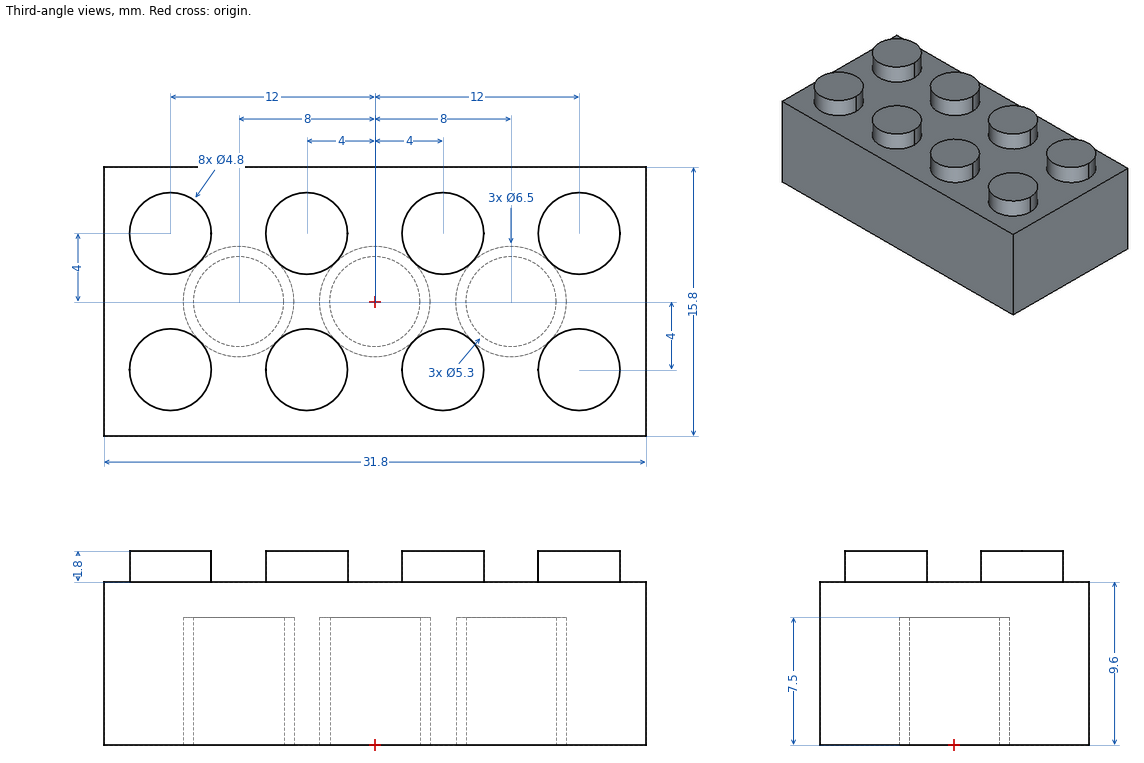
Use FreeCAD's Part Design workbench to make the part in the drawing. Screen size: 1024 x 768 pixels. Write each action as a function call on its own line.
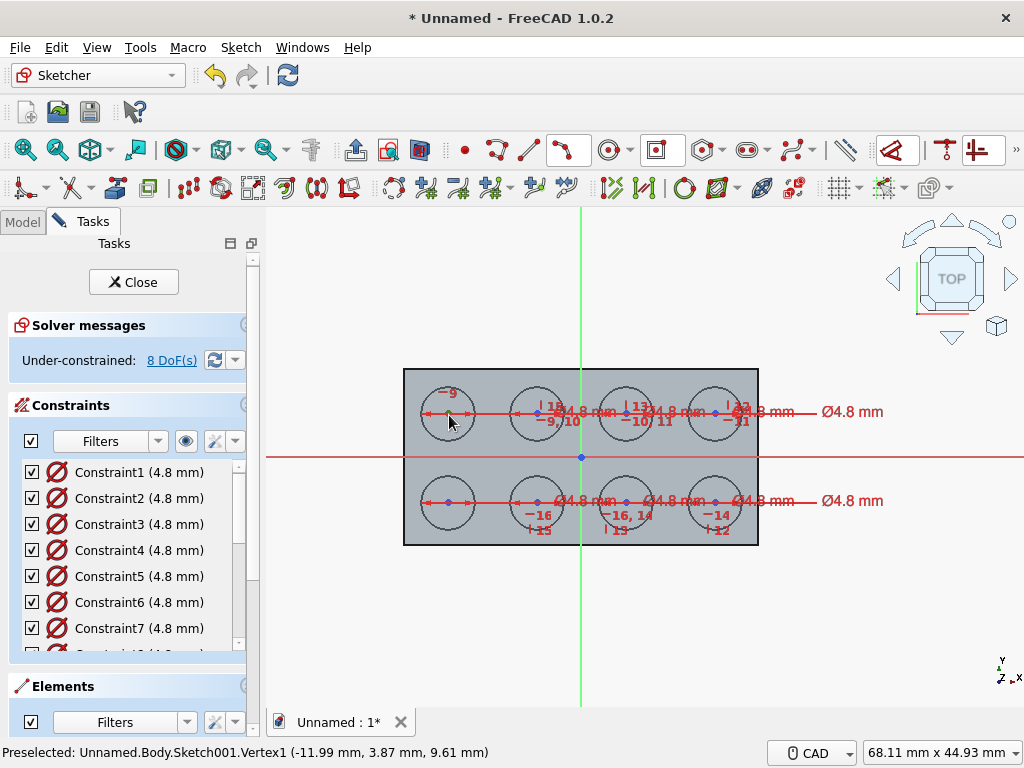
click(448, 503)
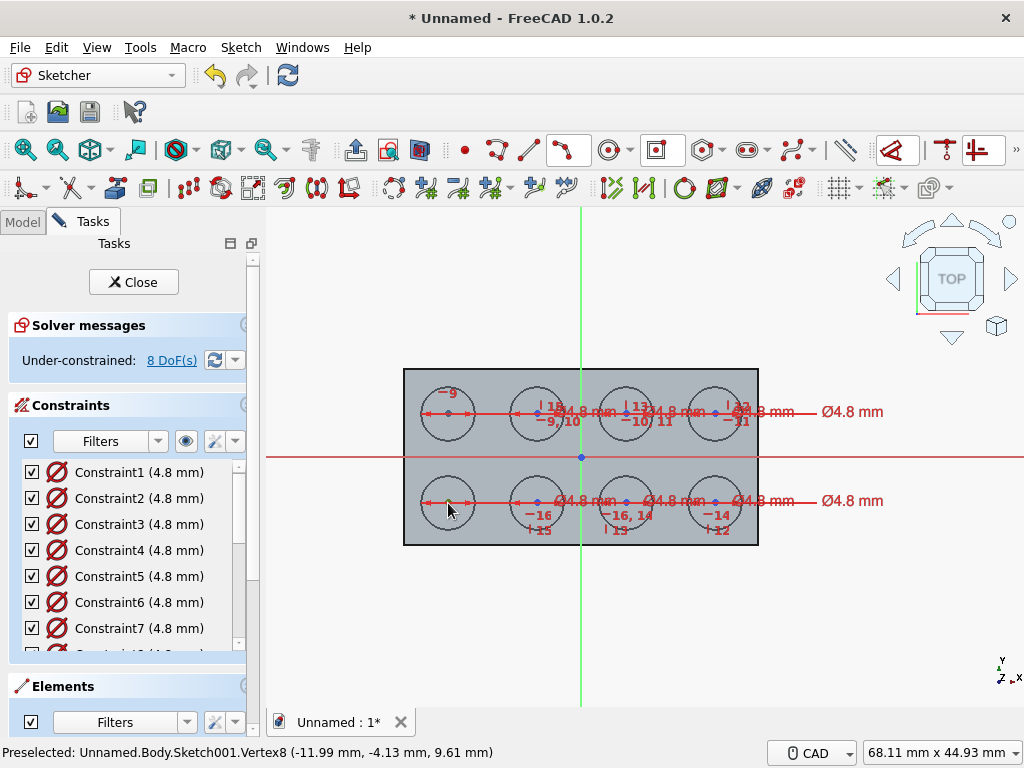
click(1000, 150)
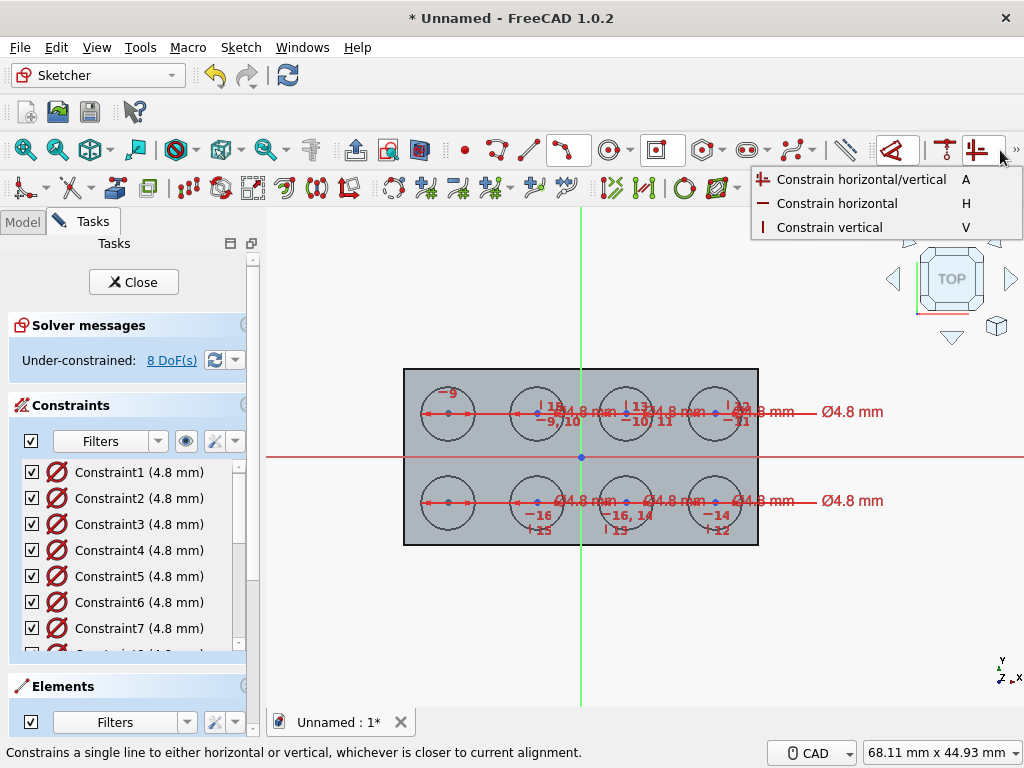
click(887, 227)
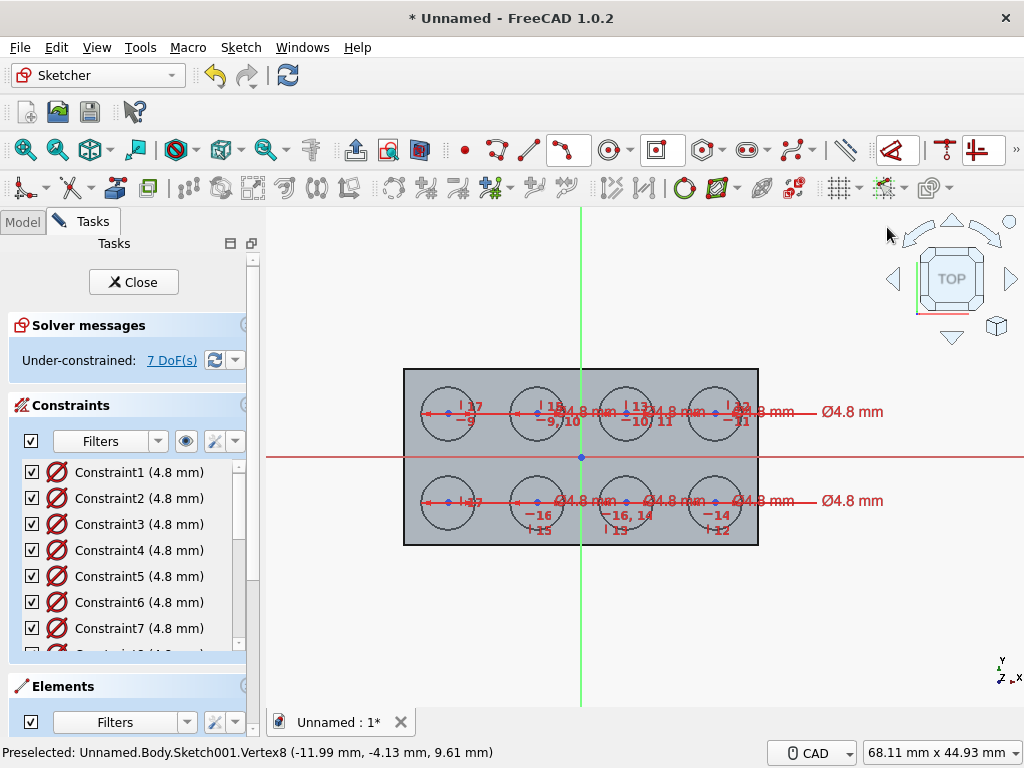
click(537, 503)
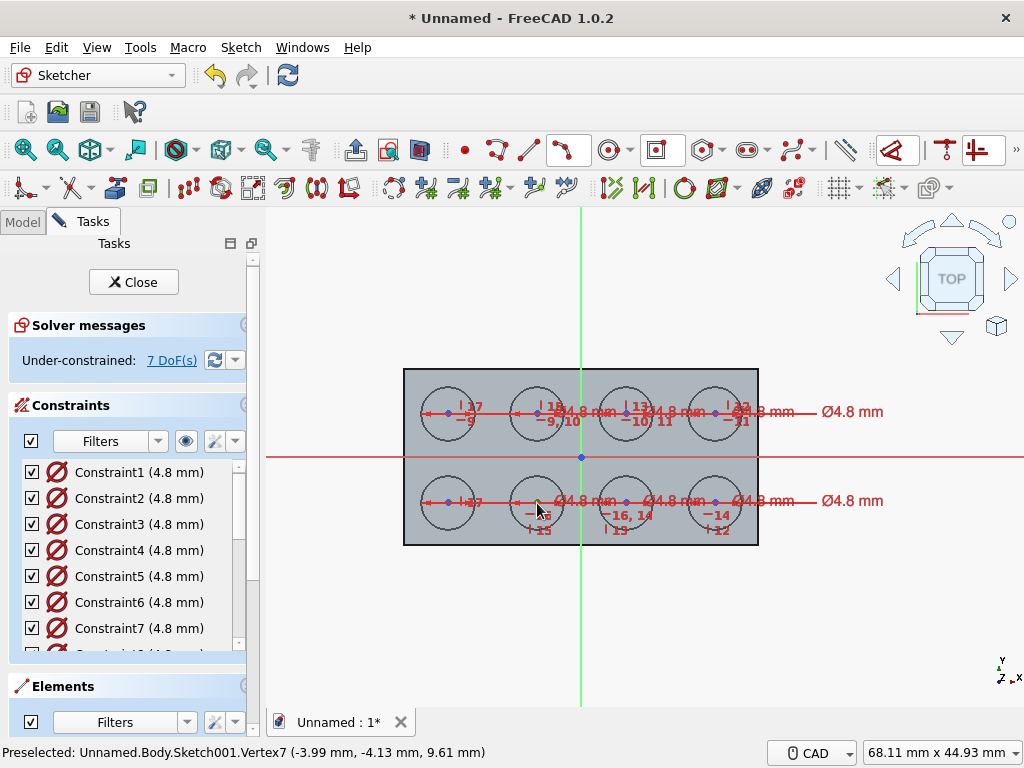
click(448, 503)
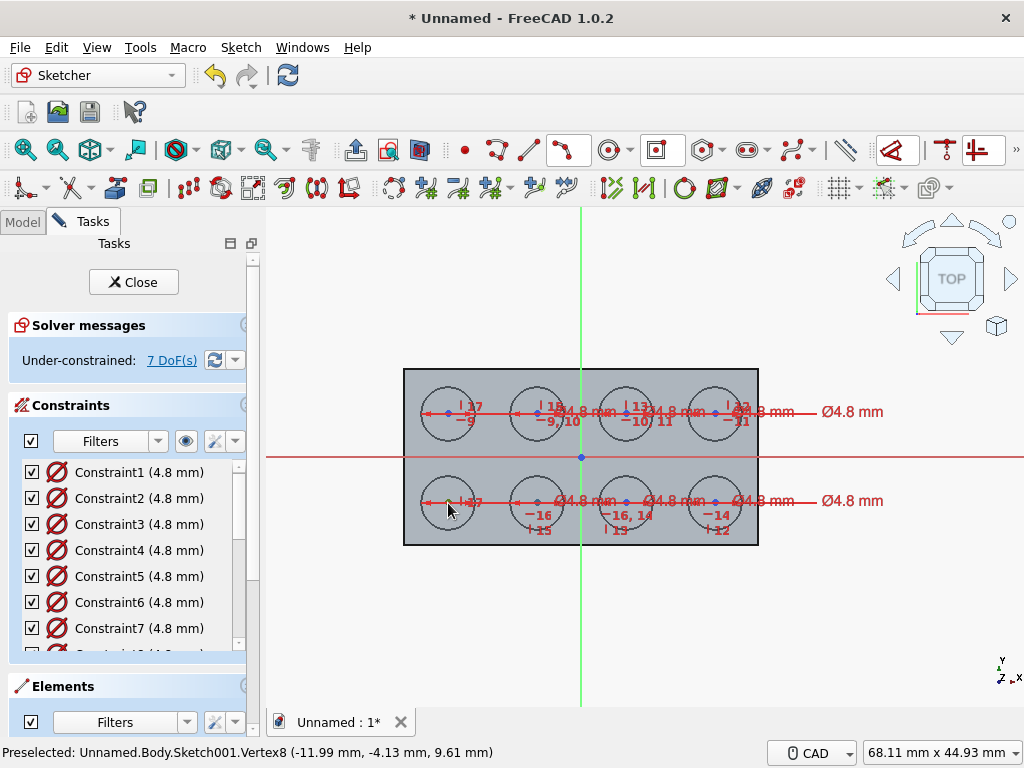
click(1000, 150)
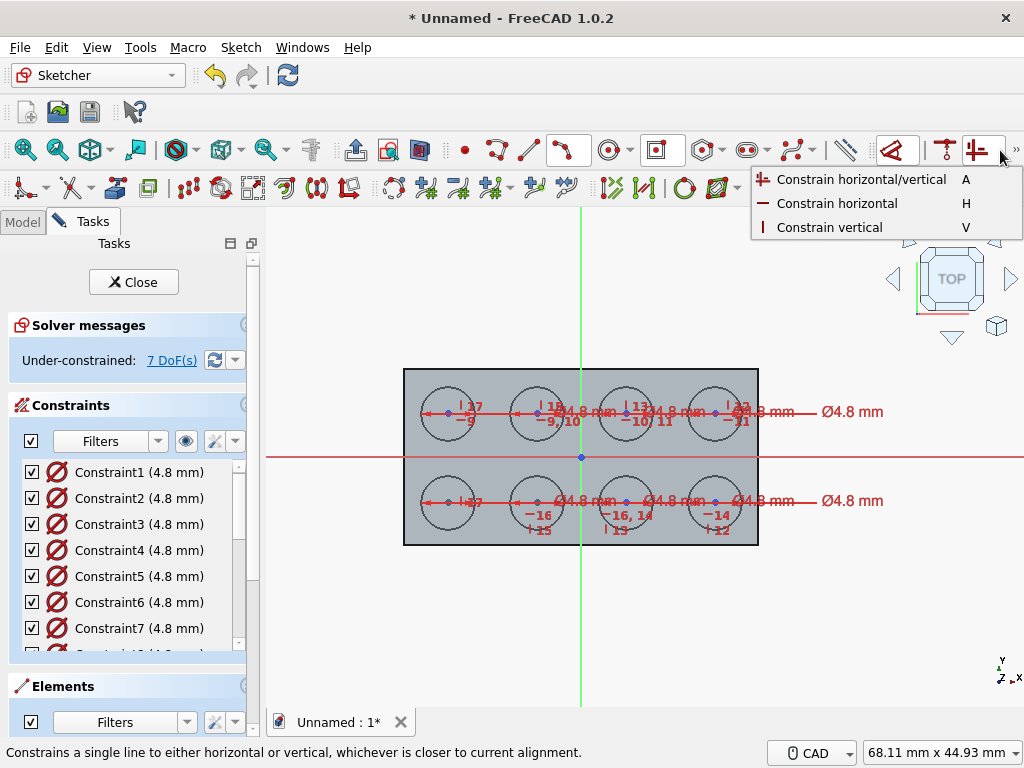
click(887, 203)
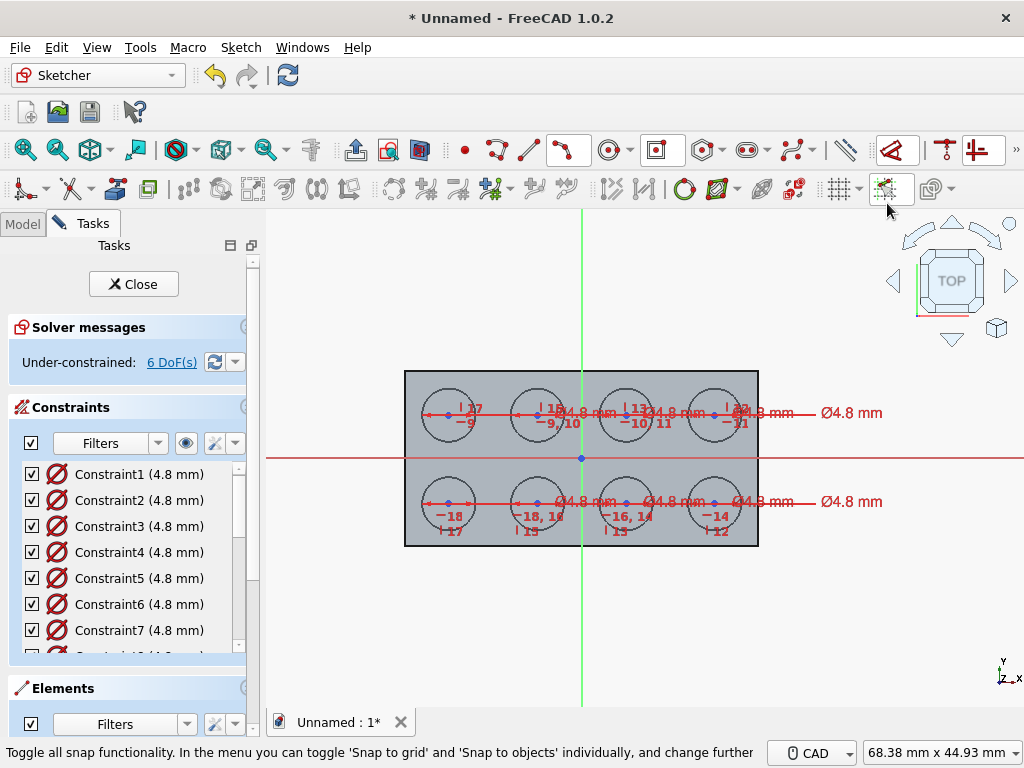
click(892, 150)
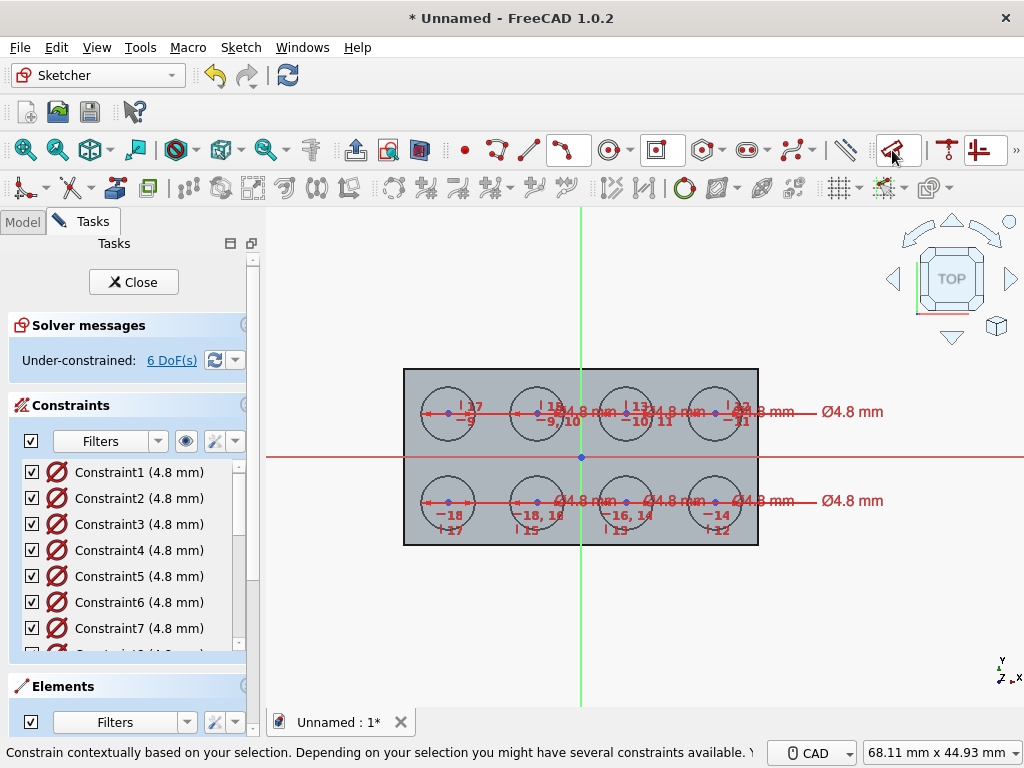
click(448, 414)
click(414, 436)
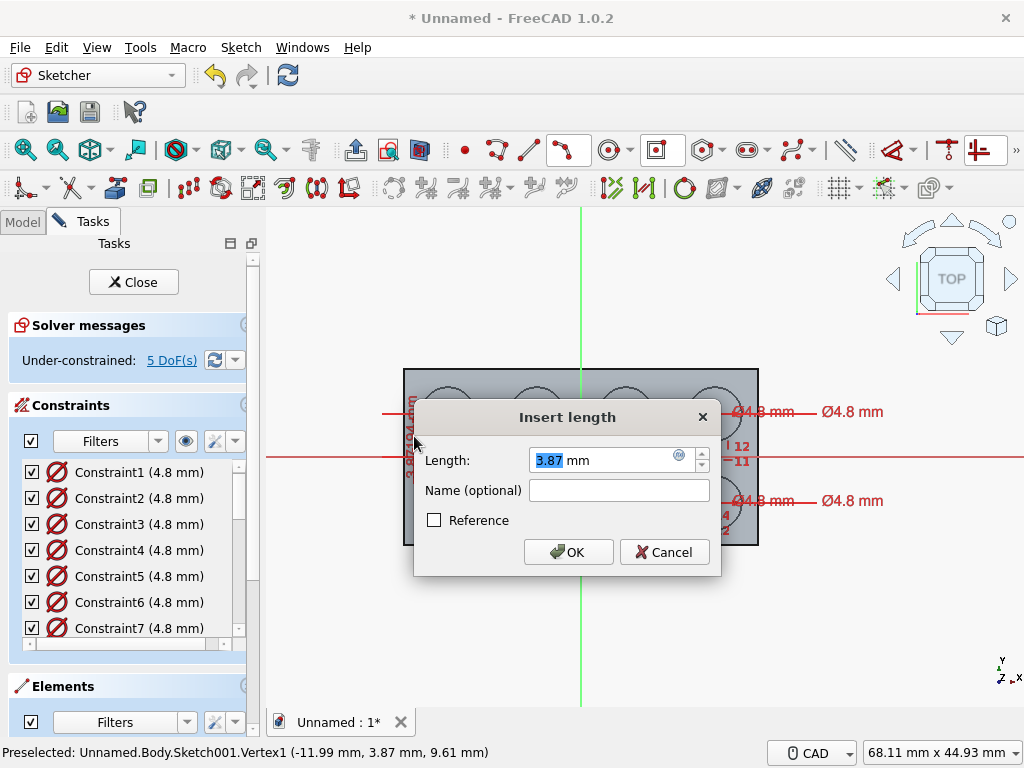
text(4)
key(Return)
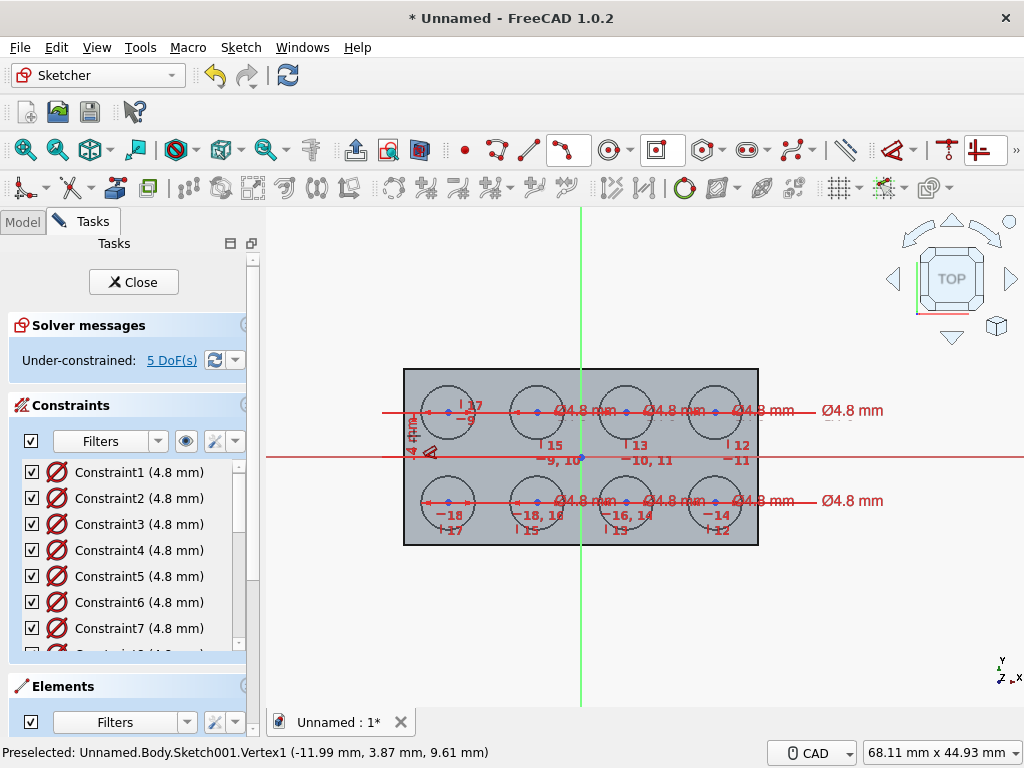
click(537, 413)
click(559, 379)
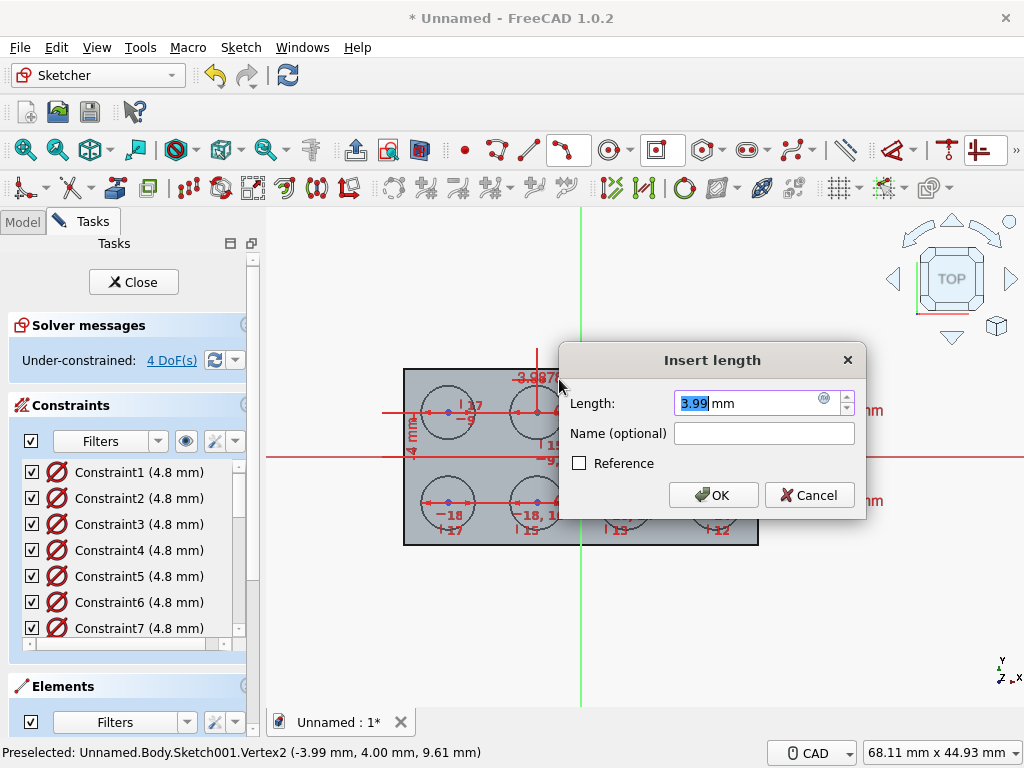
text(4)
key(Return)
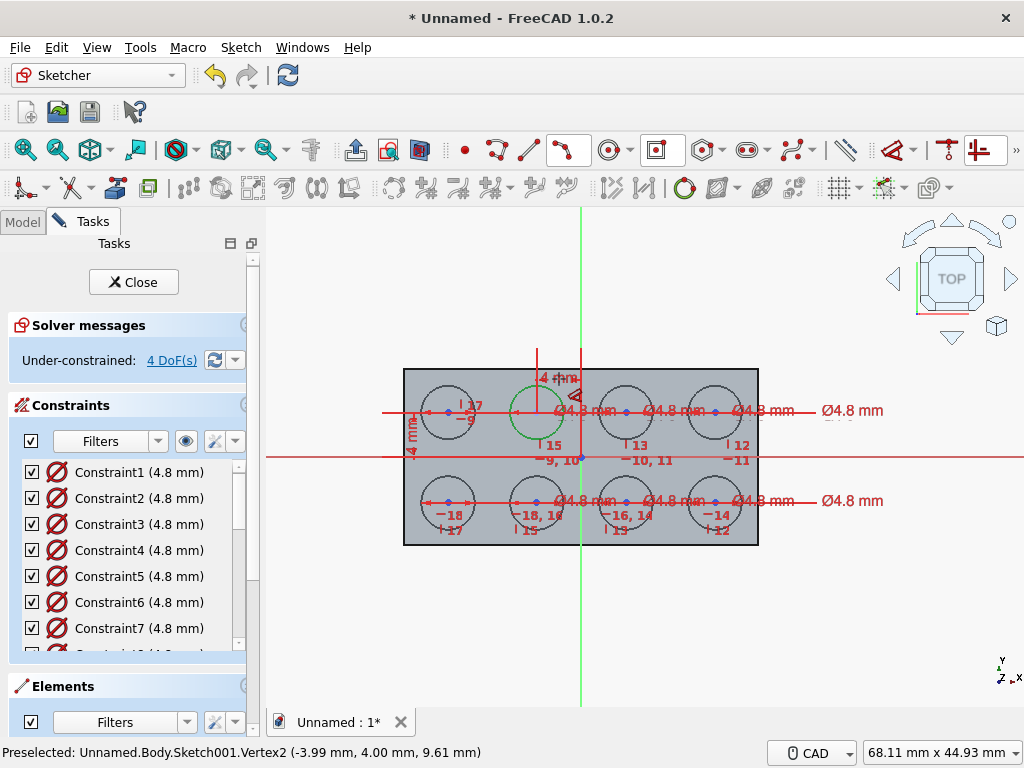
click(626, 413)
click(619, 491)